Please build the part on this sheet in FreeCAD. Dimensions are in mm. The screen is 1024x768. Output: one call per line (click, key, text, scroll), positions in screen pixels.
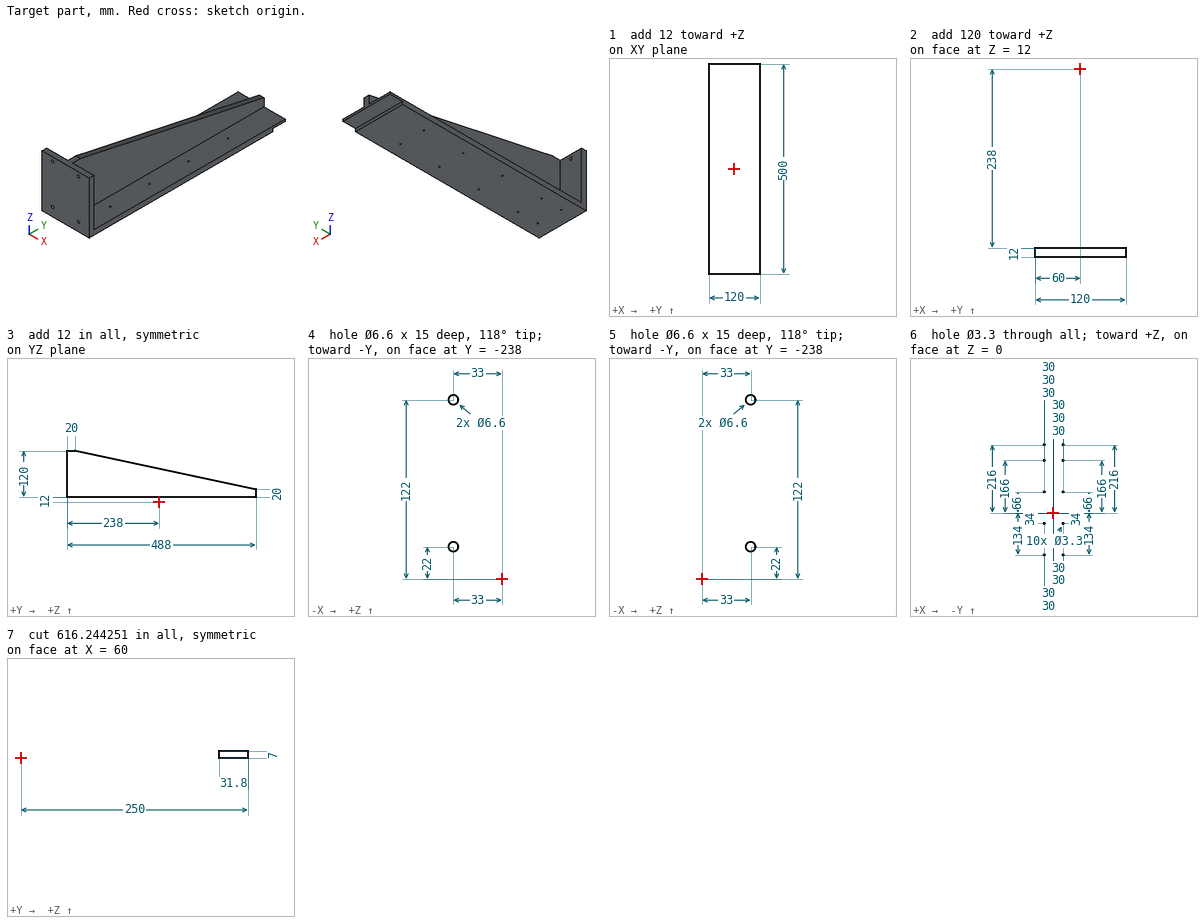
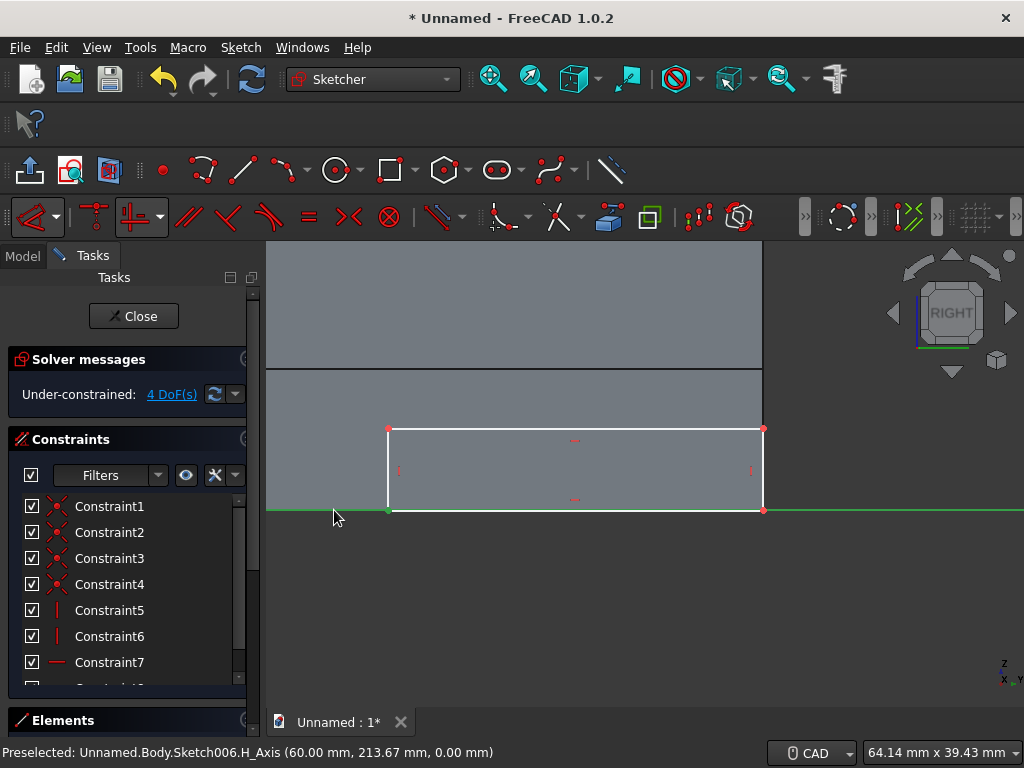
click(94, 218)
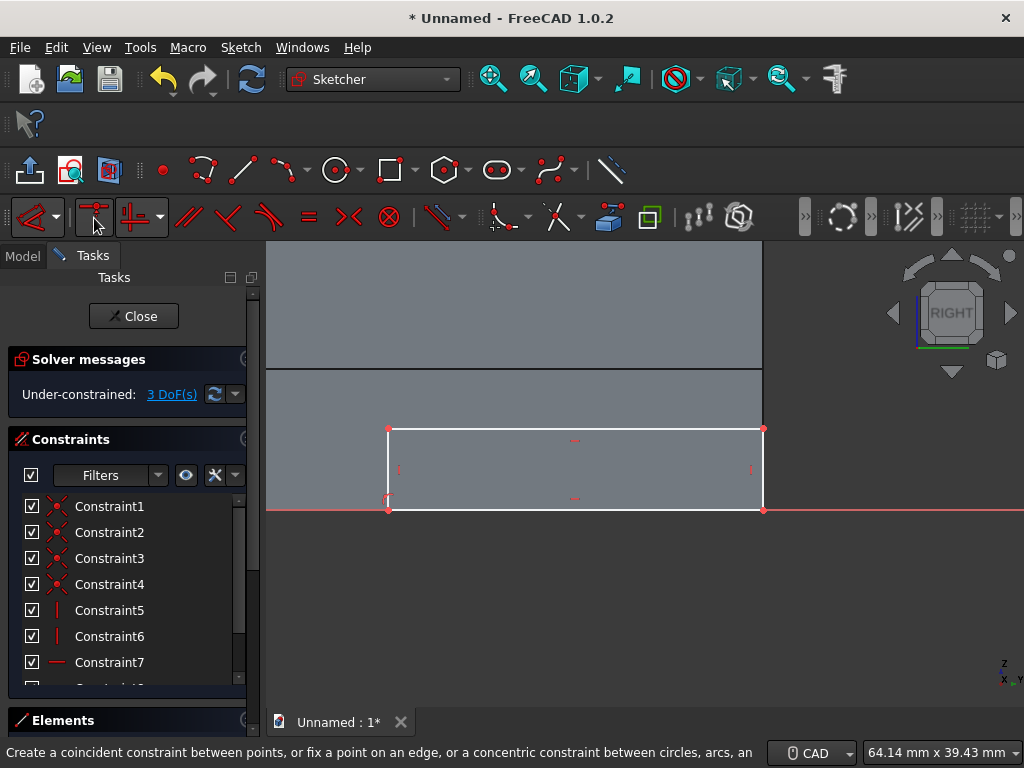
click(388, 453)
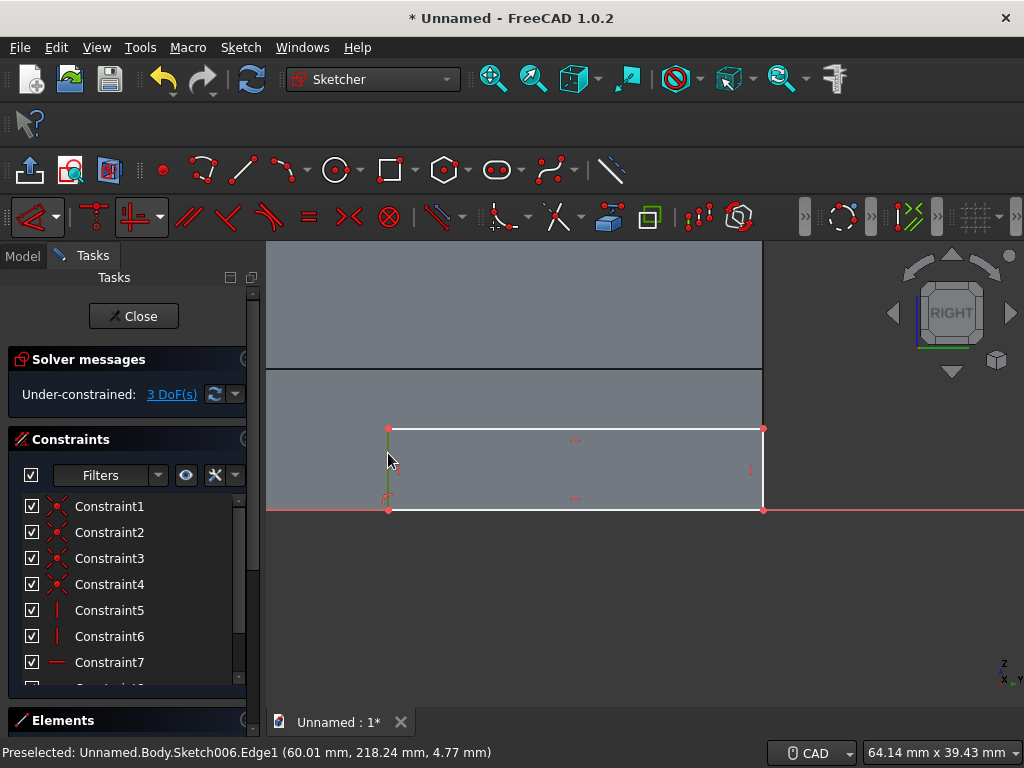
key(i)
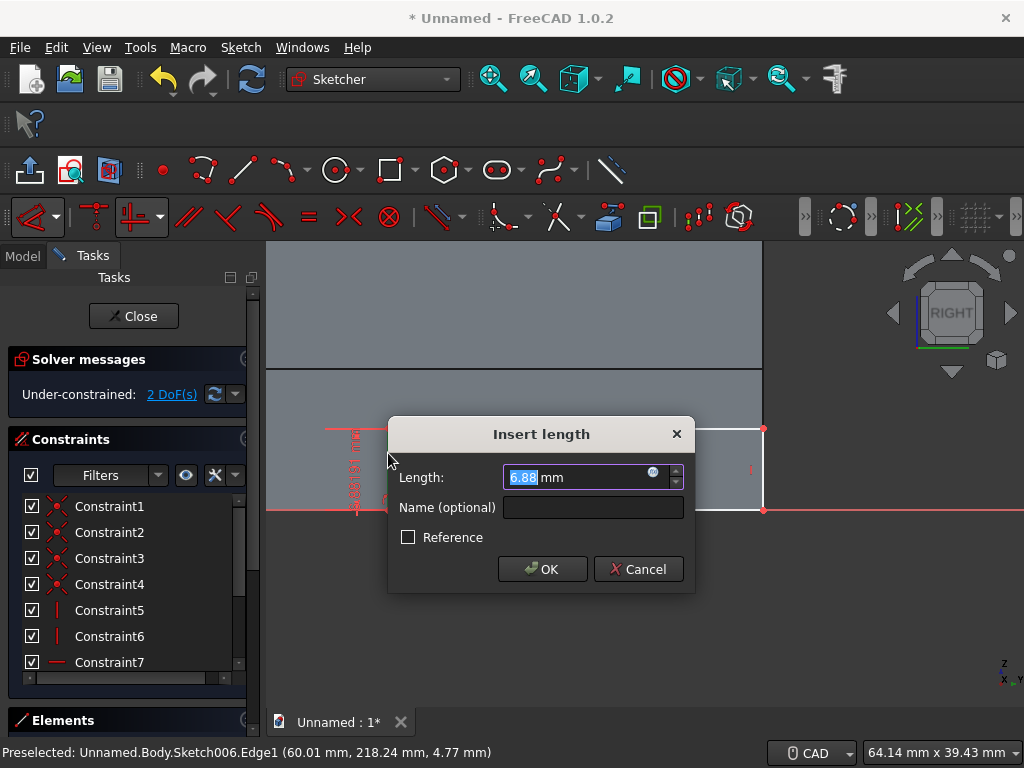
text(7)
key(Return)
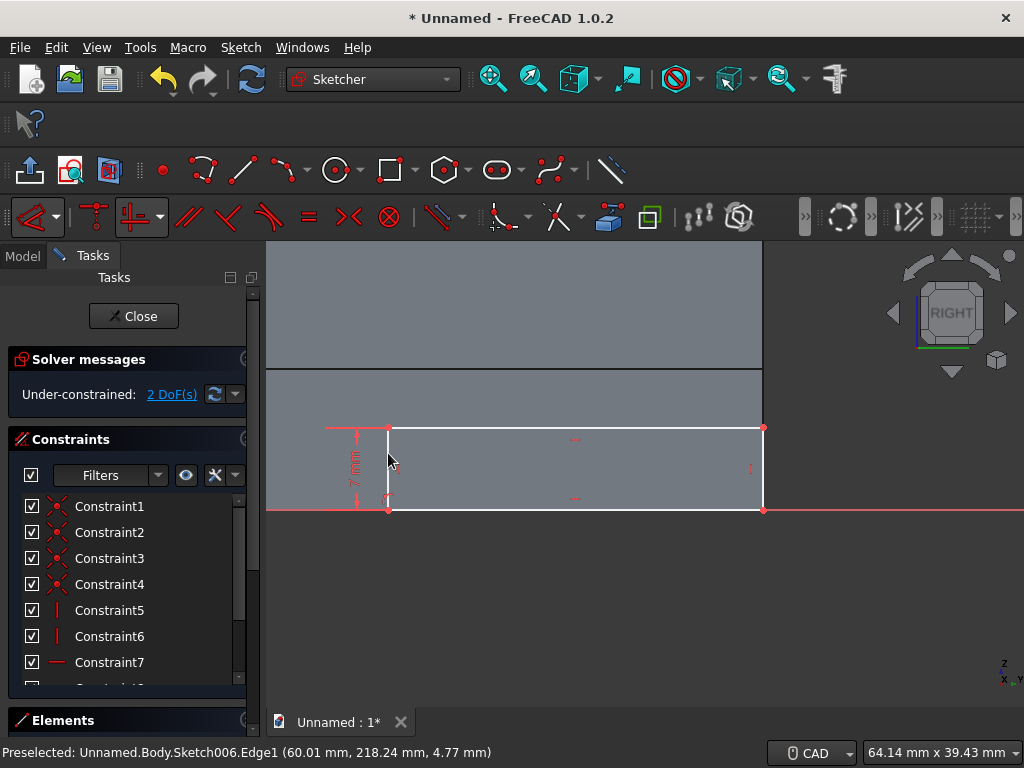
click(501, 510)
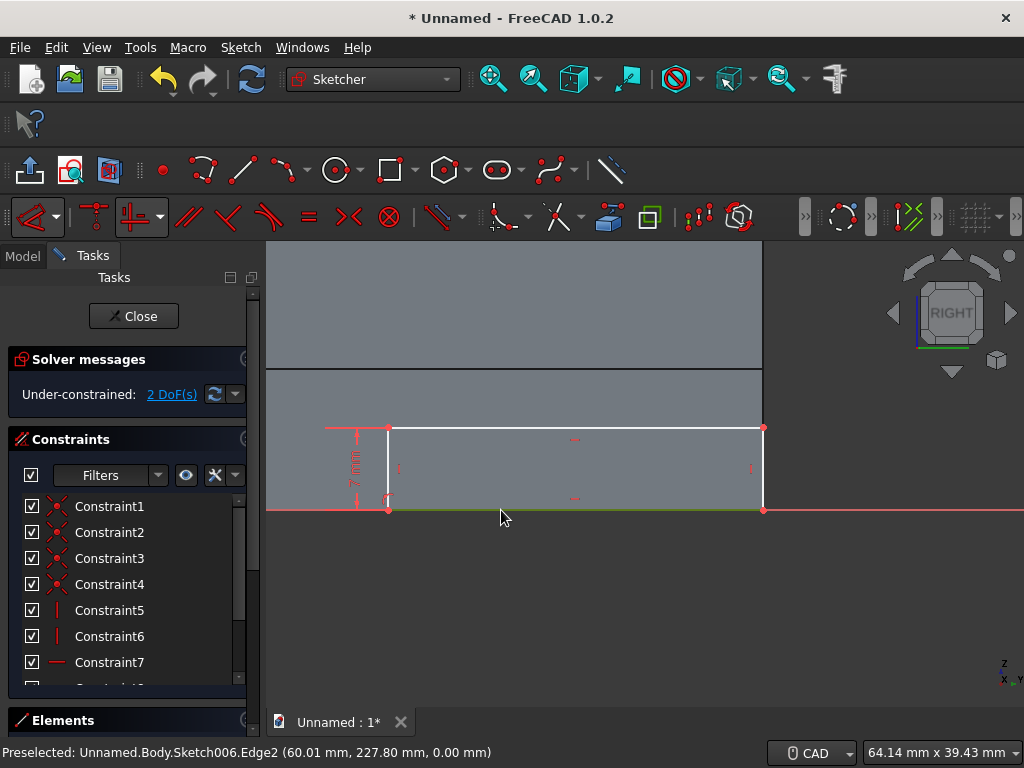
click(58, 218)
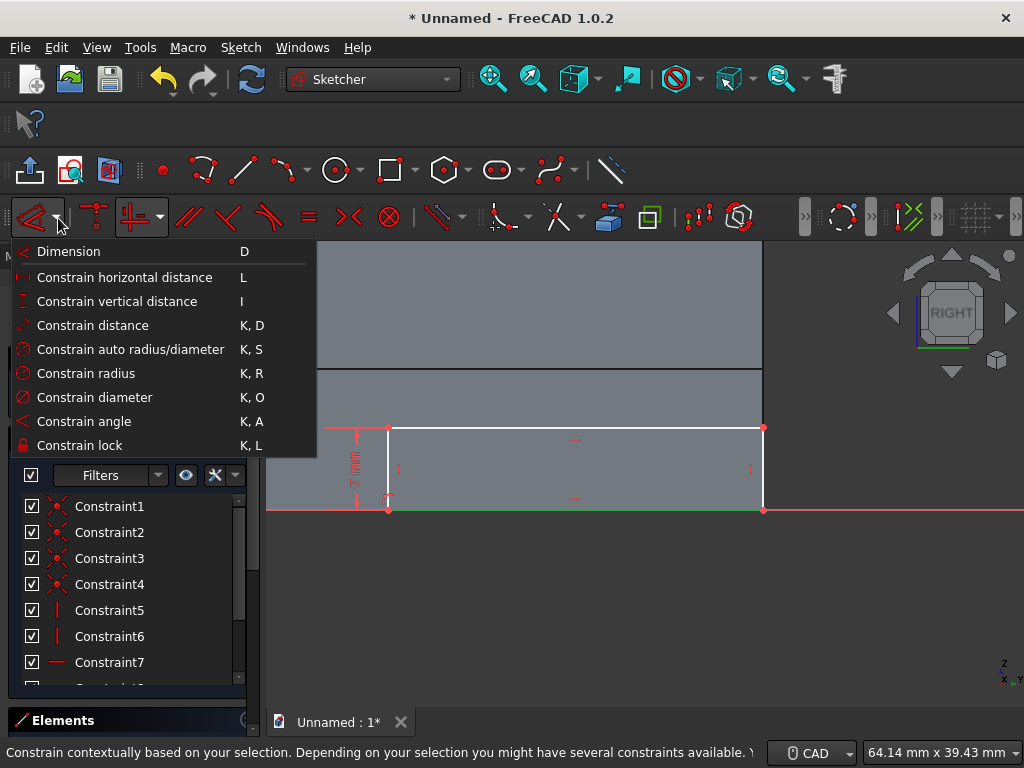
click(164, 277)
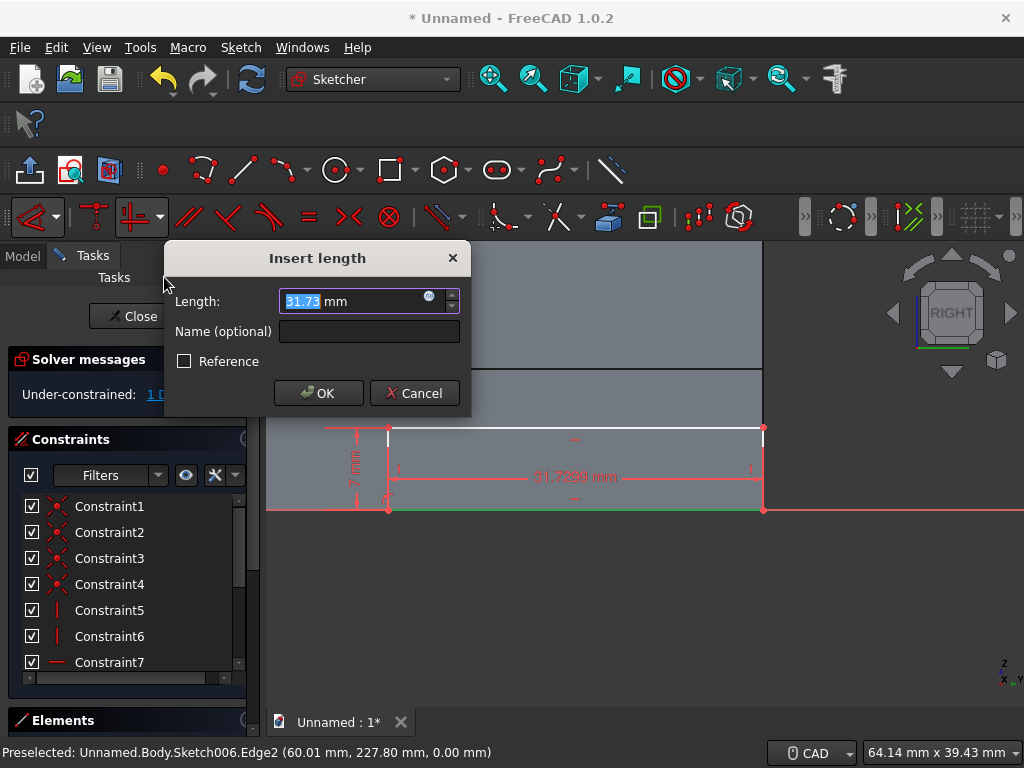
text(31.8)
key(Return)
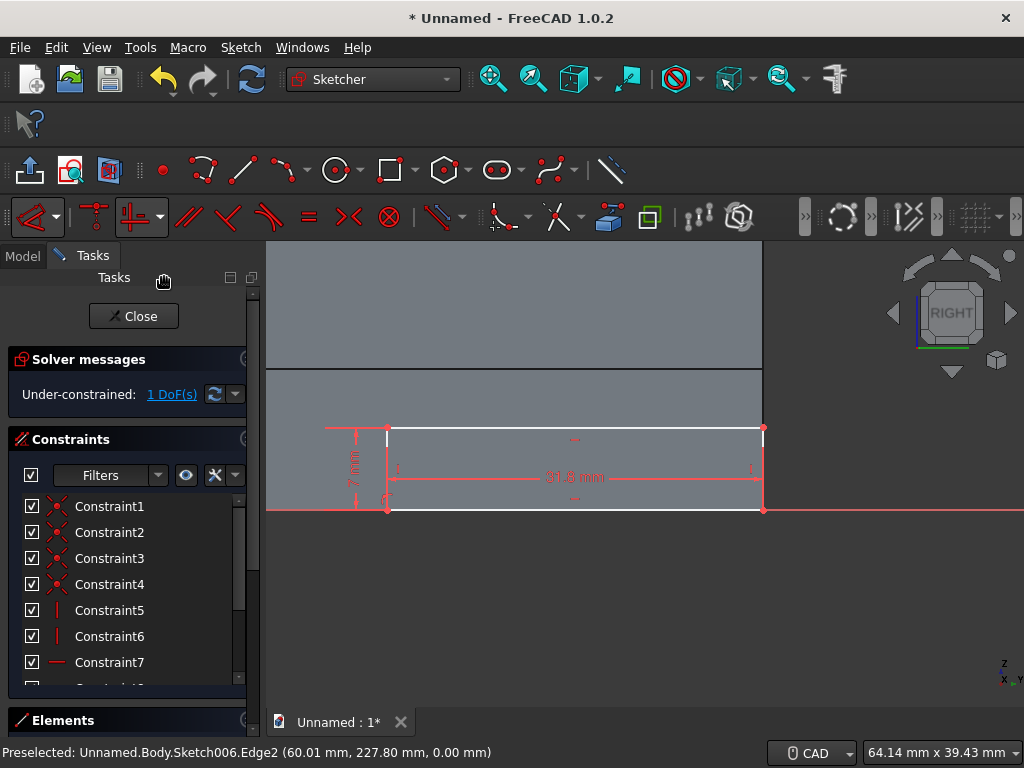
click(763, 510)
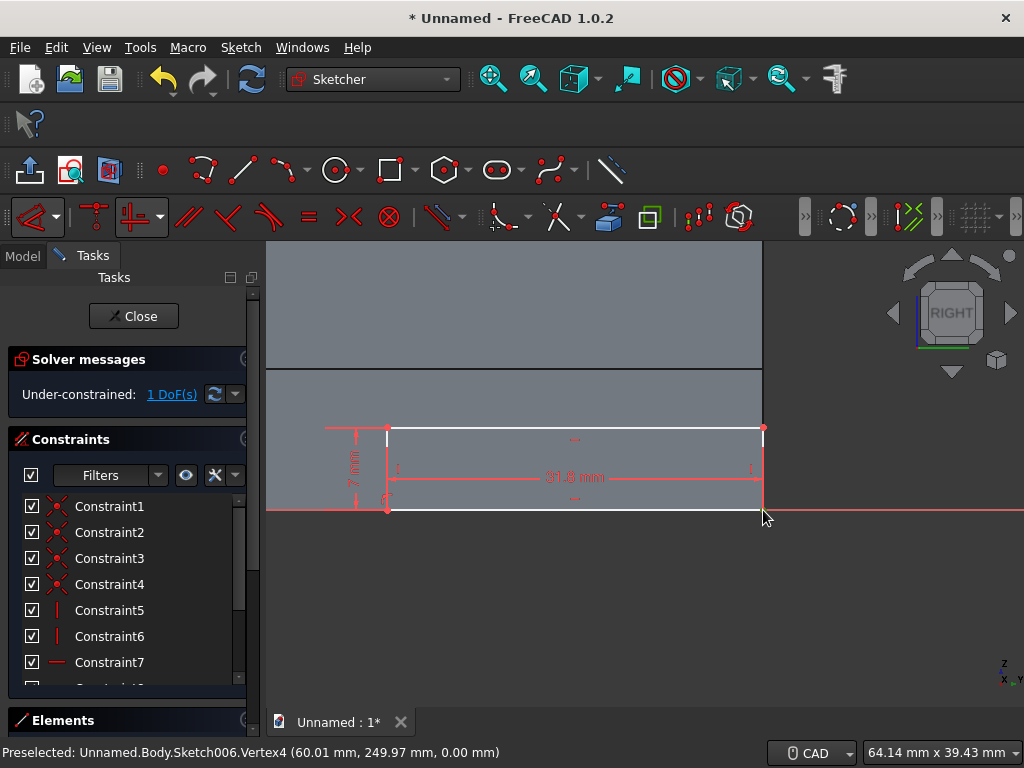
click(58, 218)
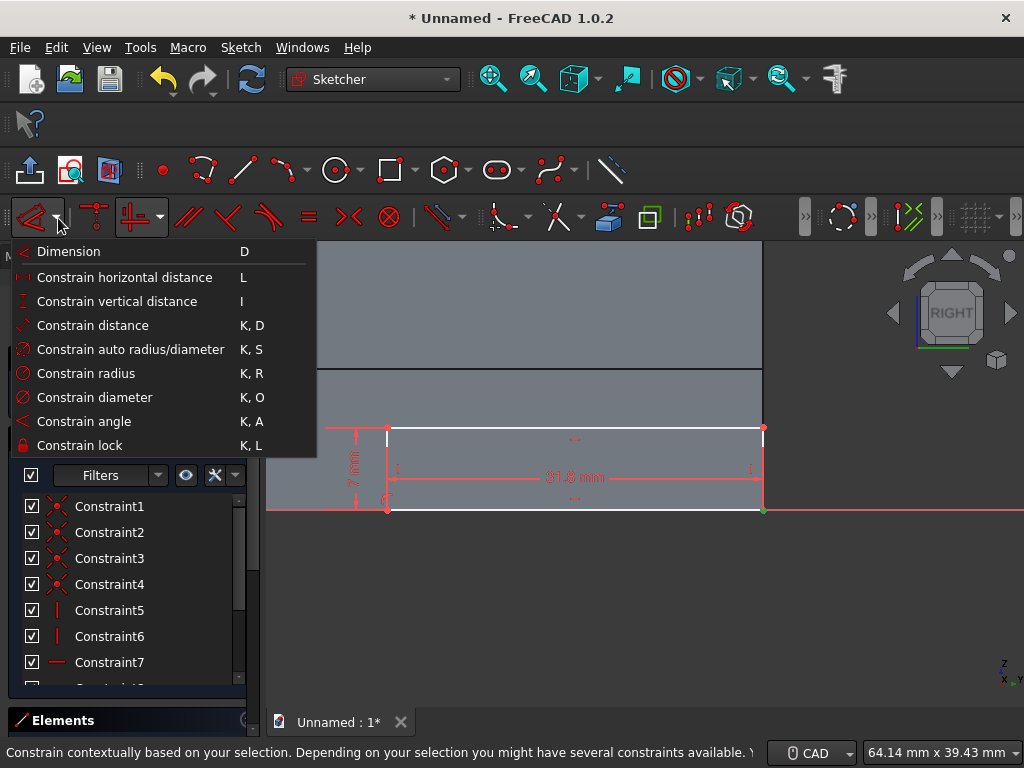
click(164, 277)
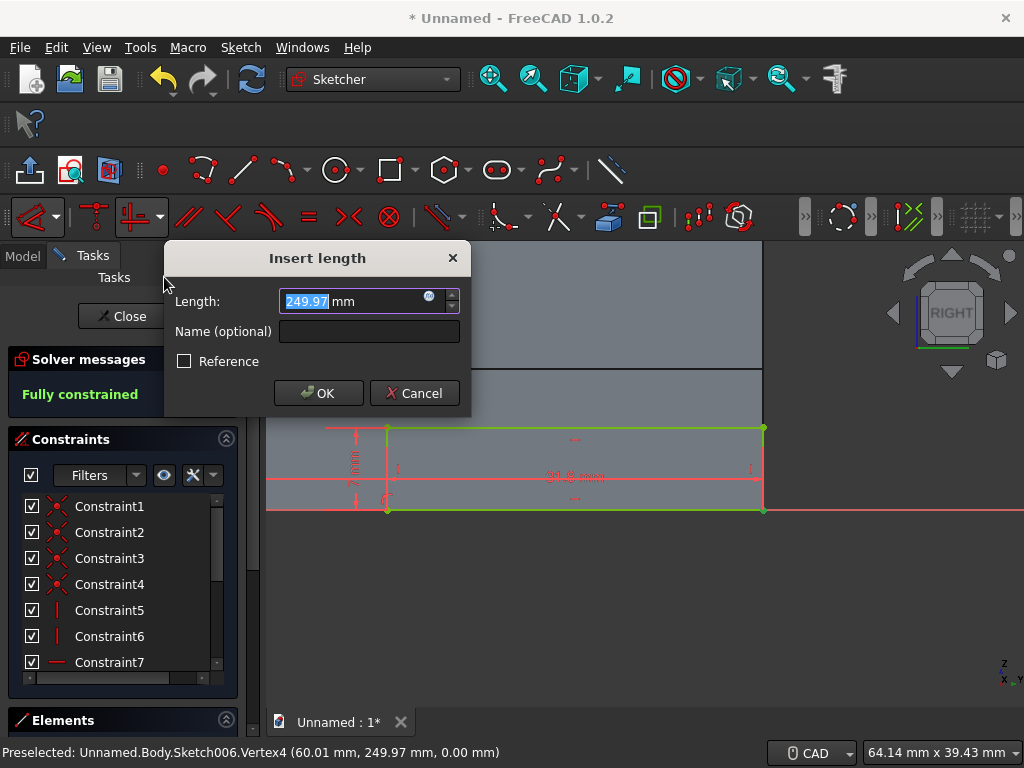
text(250)
key(Return)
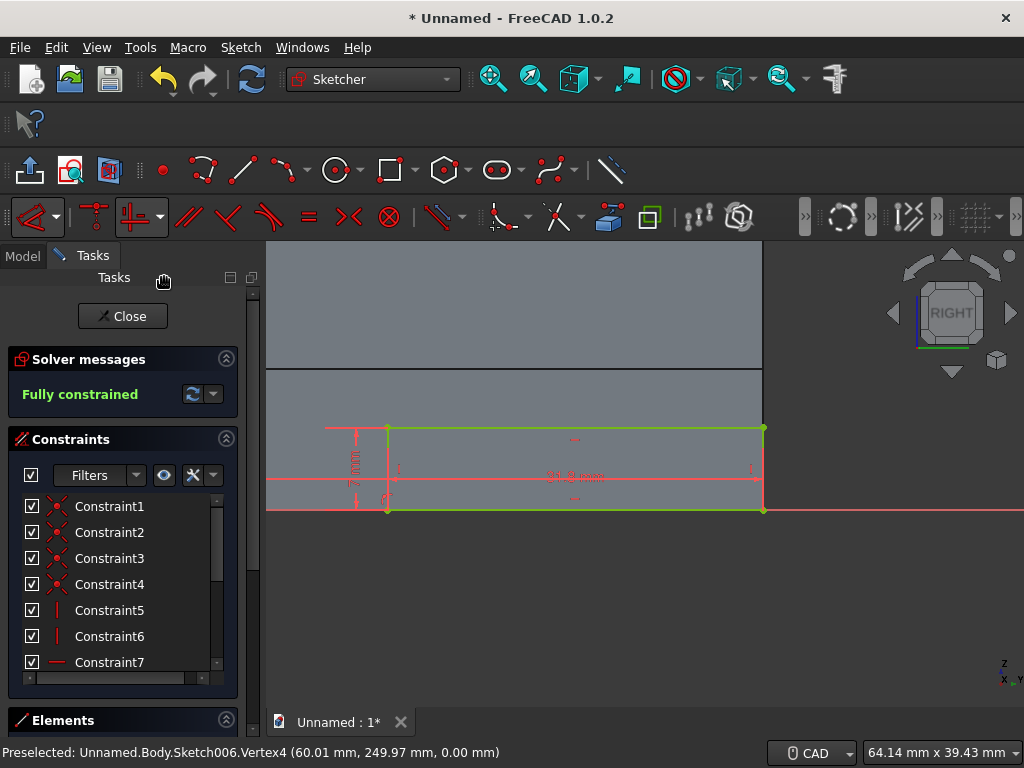
click(123, 316)